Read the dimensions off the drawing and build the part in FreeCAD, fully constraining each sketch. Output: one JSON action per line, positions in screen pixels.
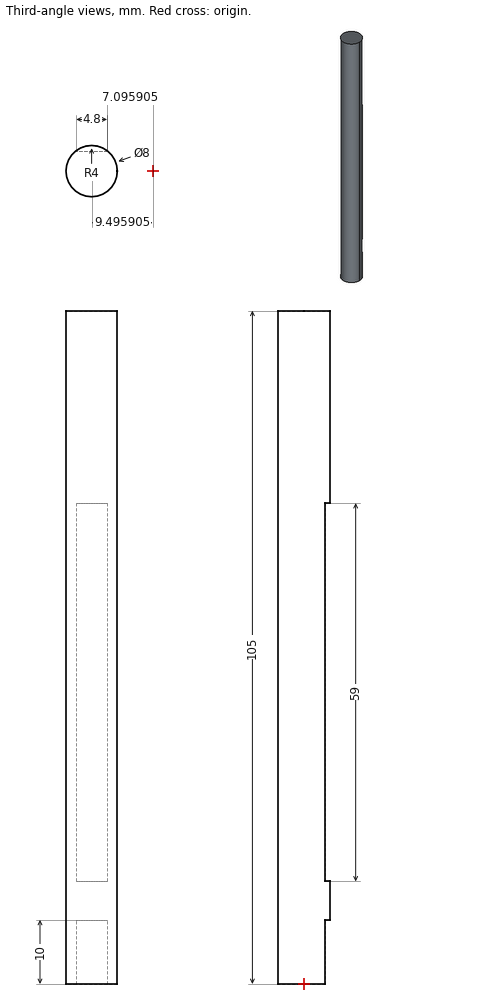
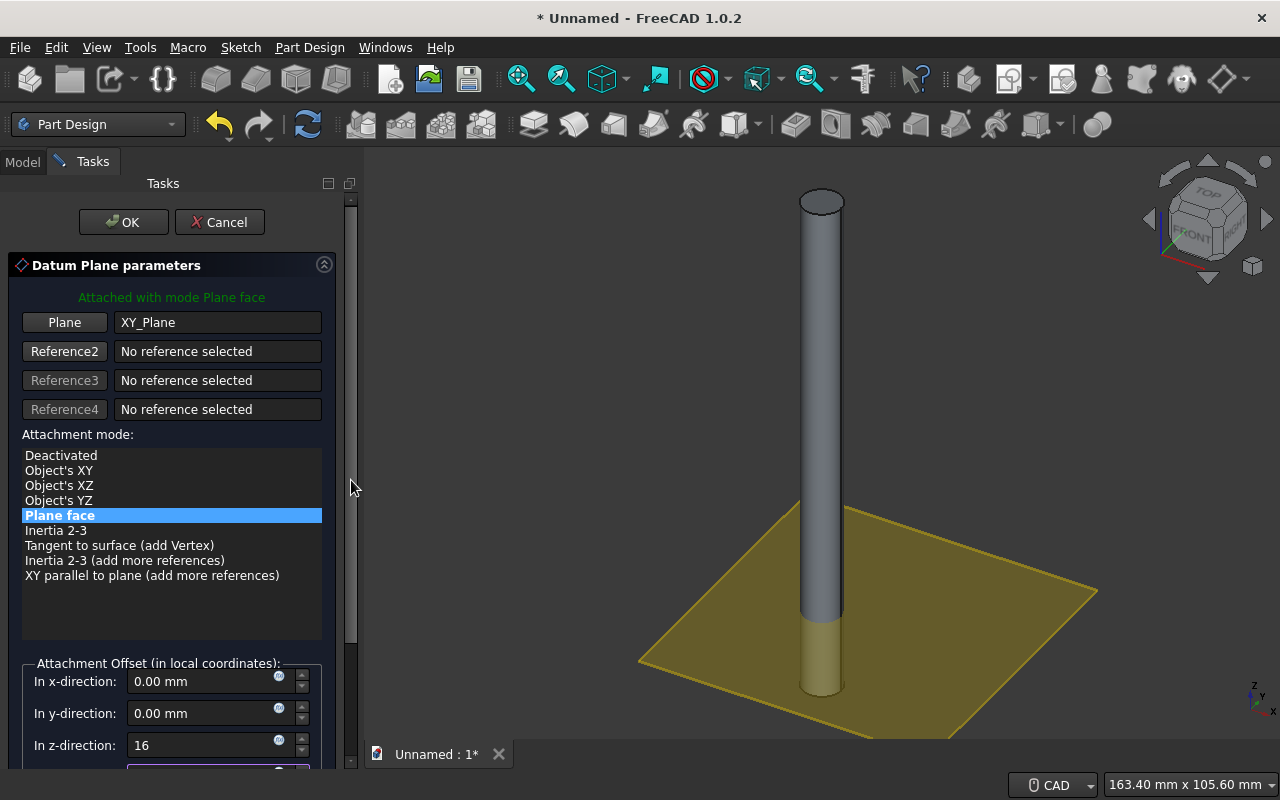
{"action": "left_click", "coordinate": [124, 222]}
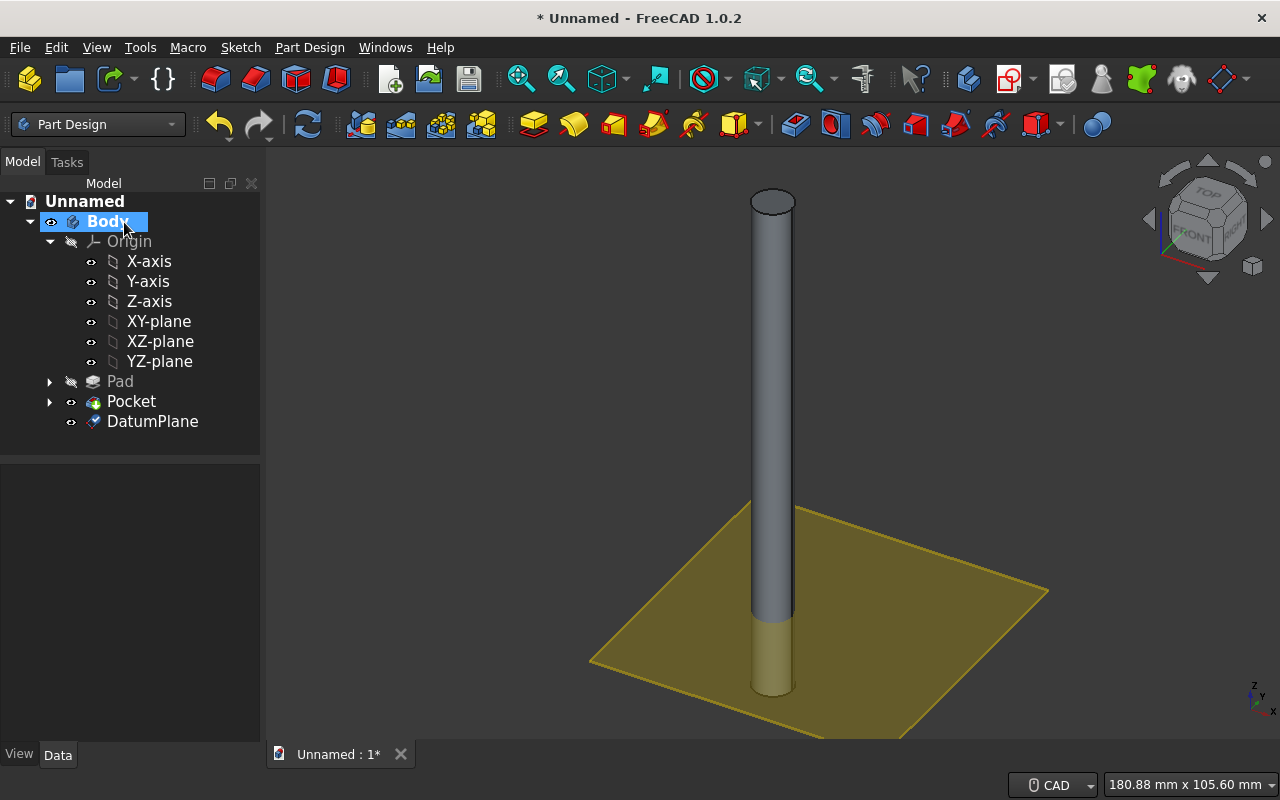
{"action": "left_click", "coordinate": [116, 422]}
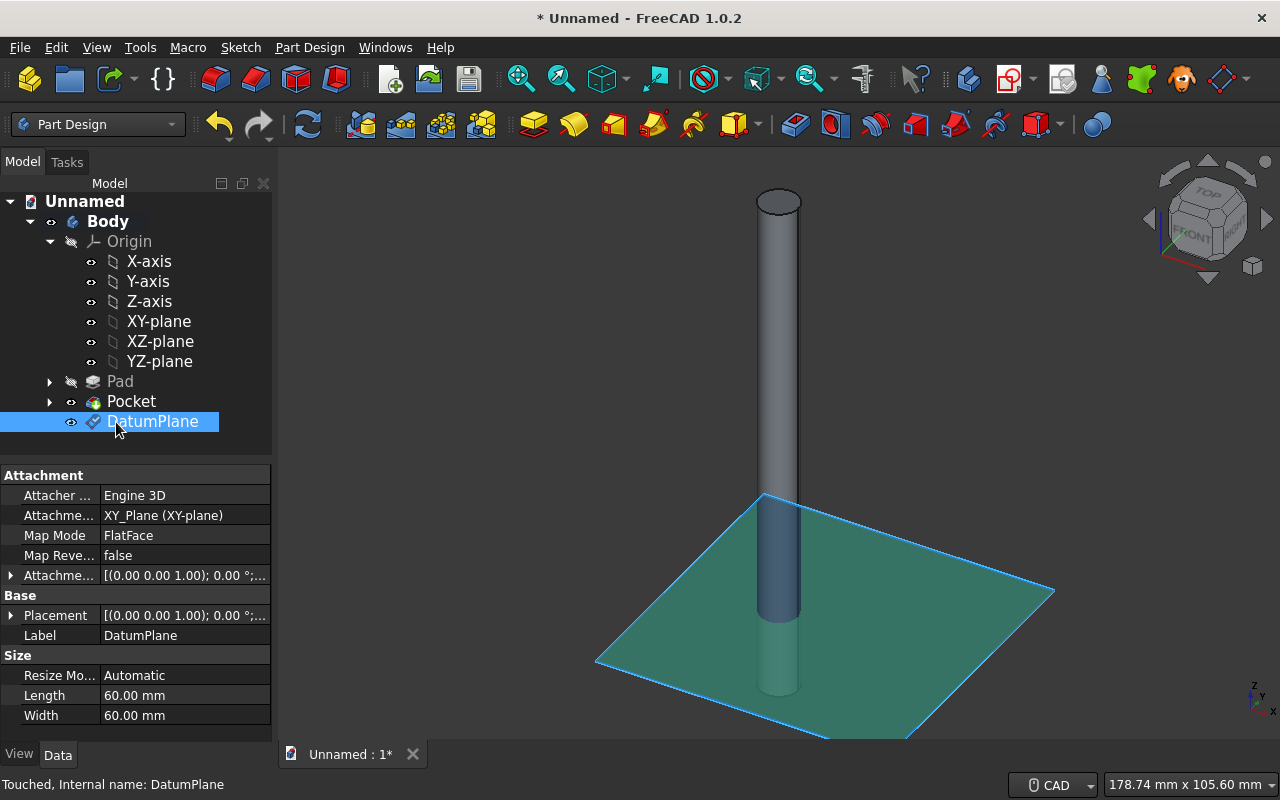
{"action": "left_click", "coordinate": [1010, 80]}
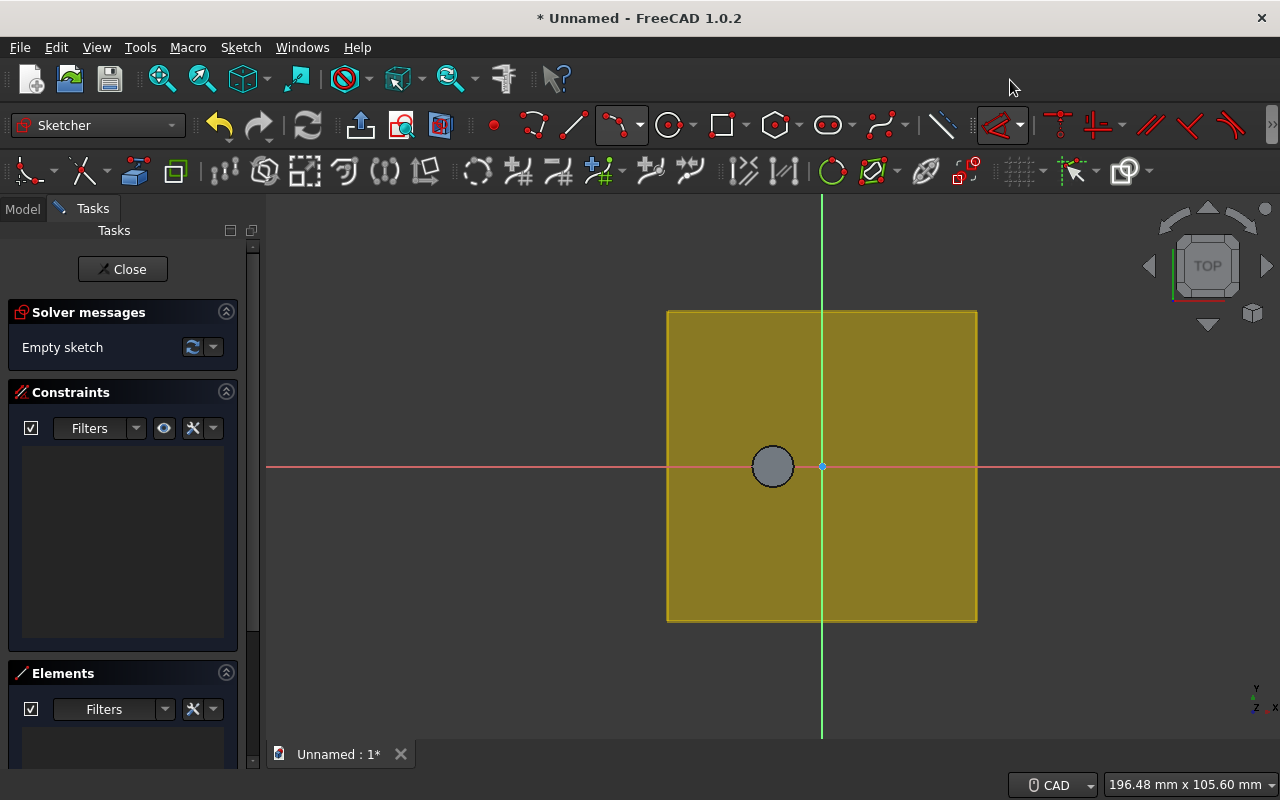
{"action": "left_click", "coordinate": [442, 126]}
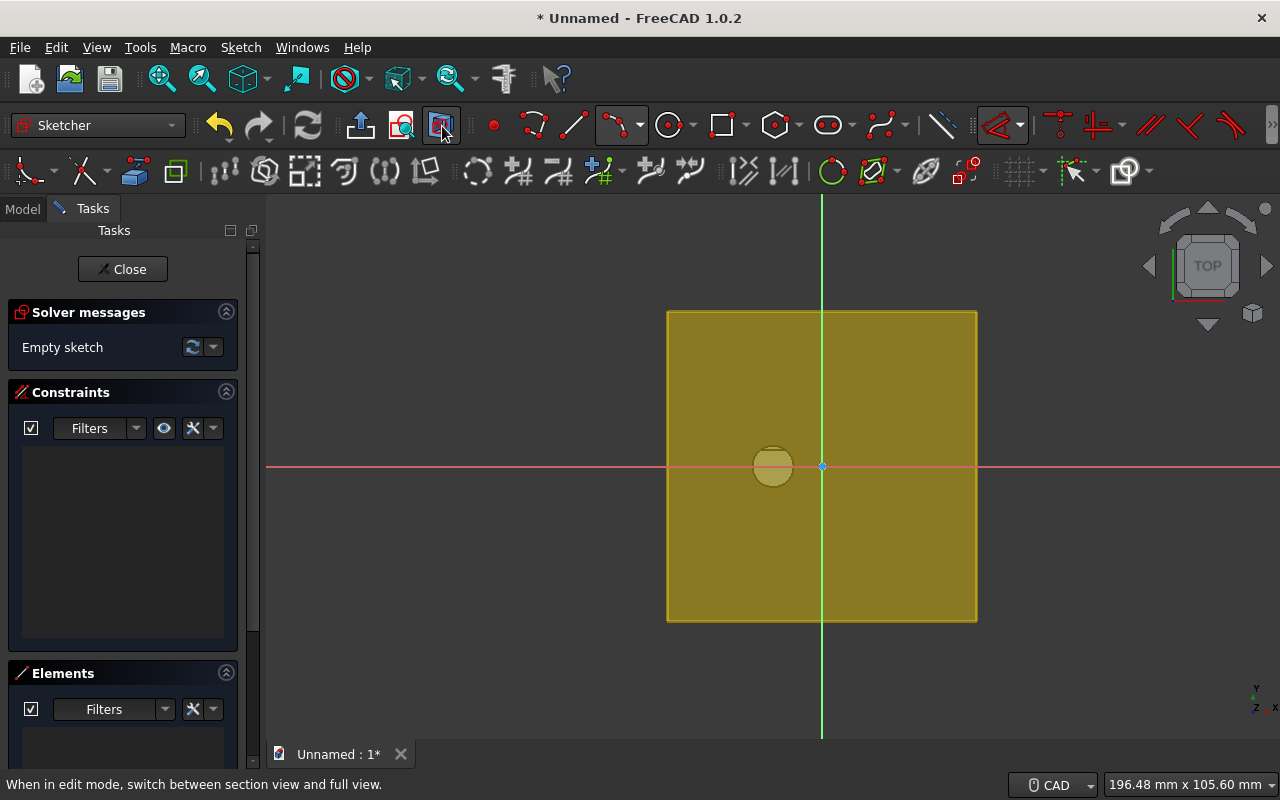
{"action": "scroll", "coordinate": [802, 455], "scroll_direction": "up", "scroll_amount": 11}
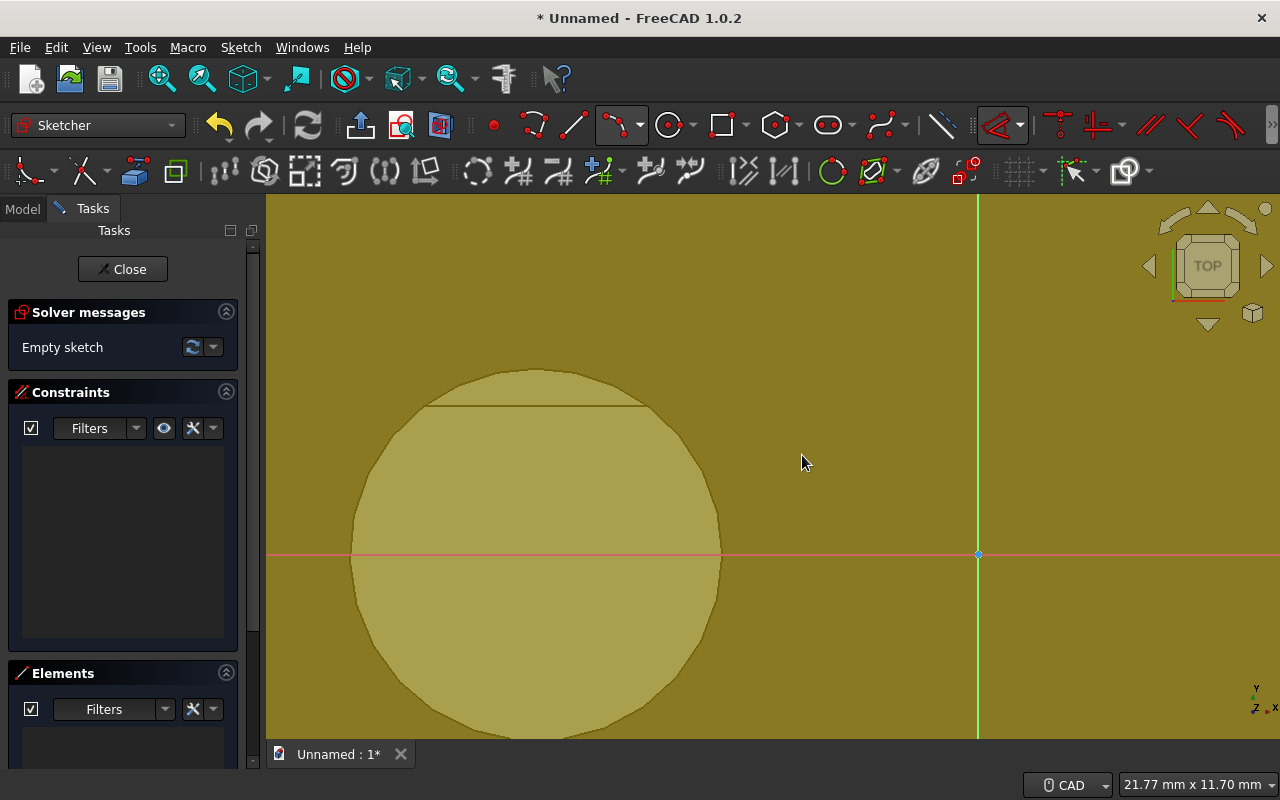
{"action": "left_click", "coordinate": [574, 126]}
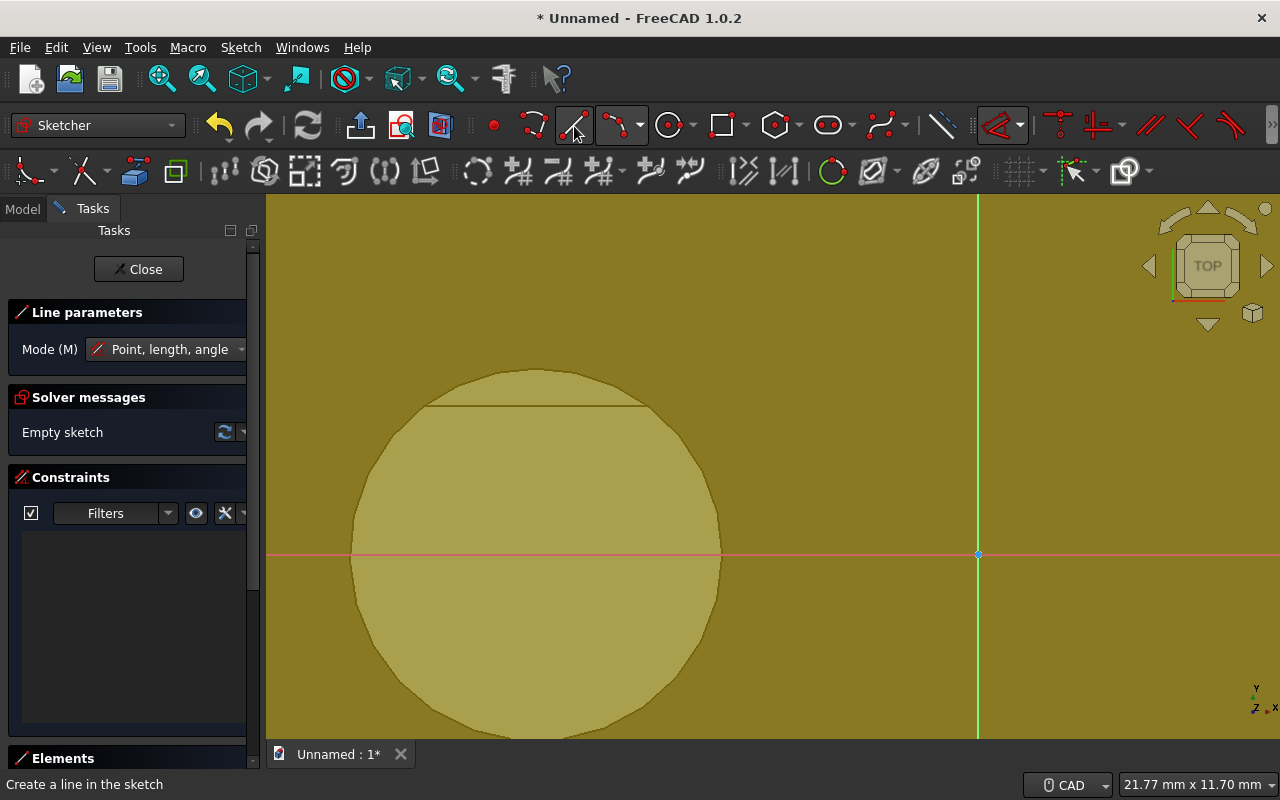
{"action": "left_click", "coordinate": [648, 406]}
{"action": "left_click", "coordinate": [424, 406]}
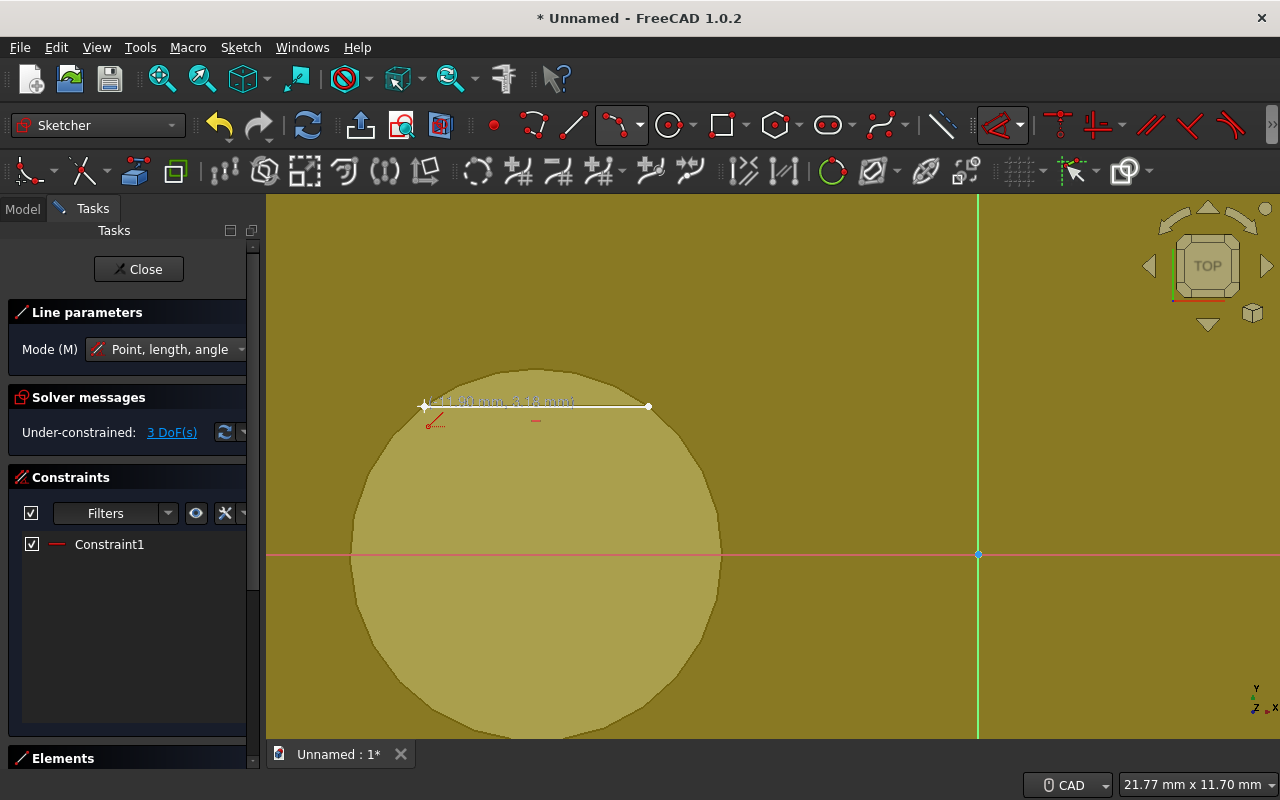
{"action": "key", "text": "g 3 a"}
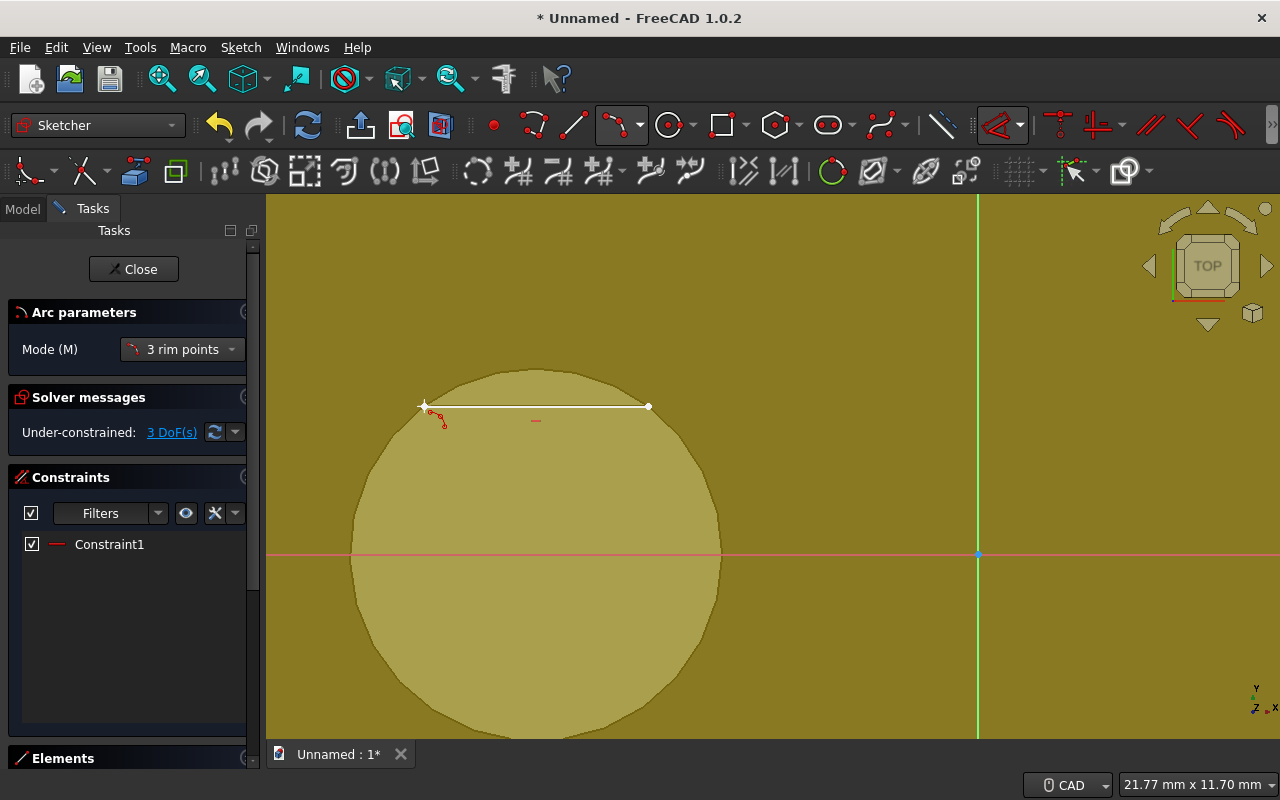
{"action": "left_click", "coordinate": [424, 407]}
{"action": "left_click", "coordinate": [648, 407]}
{"action": "left_click", "coordinate": [536, 369]}
{"action": "key", "text": "Escape"}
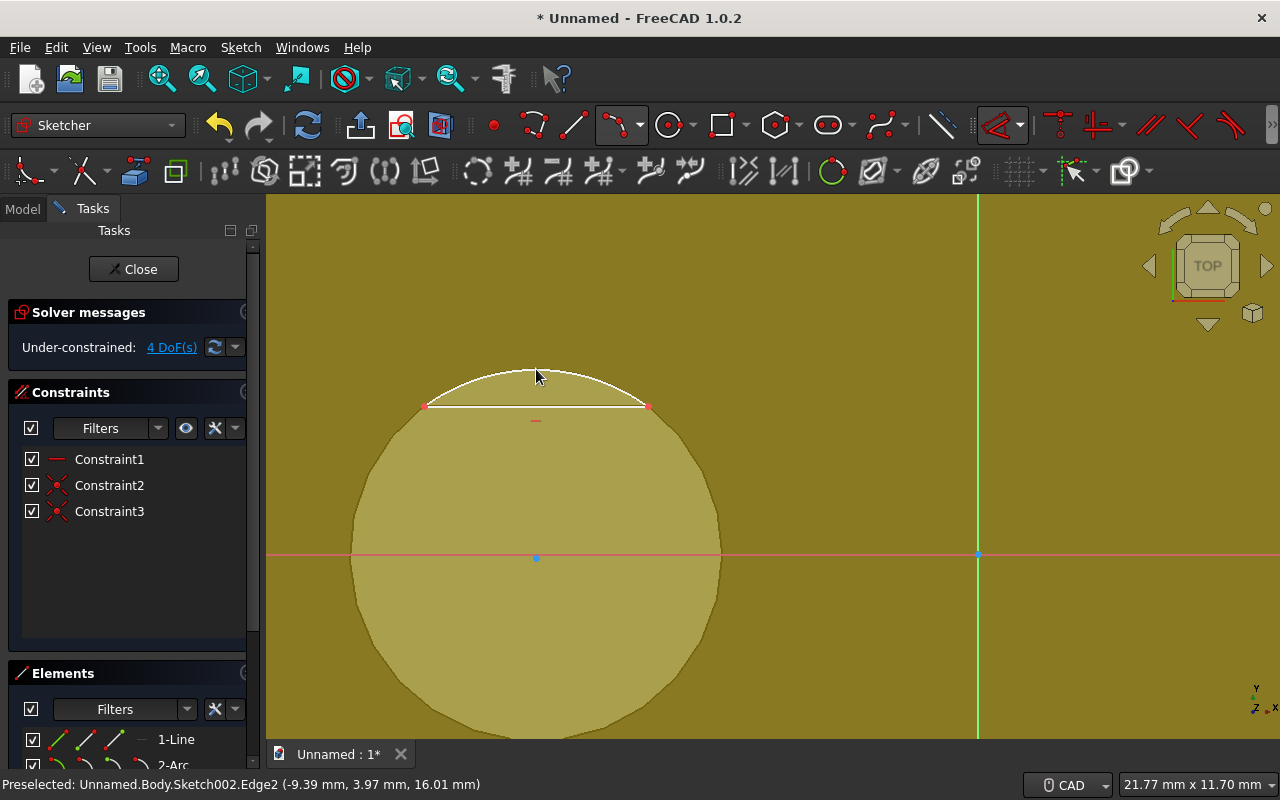
{"action": "left_click", "coordinate": [536, 558]}